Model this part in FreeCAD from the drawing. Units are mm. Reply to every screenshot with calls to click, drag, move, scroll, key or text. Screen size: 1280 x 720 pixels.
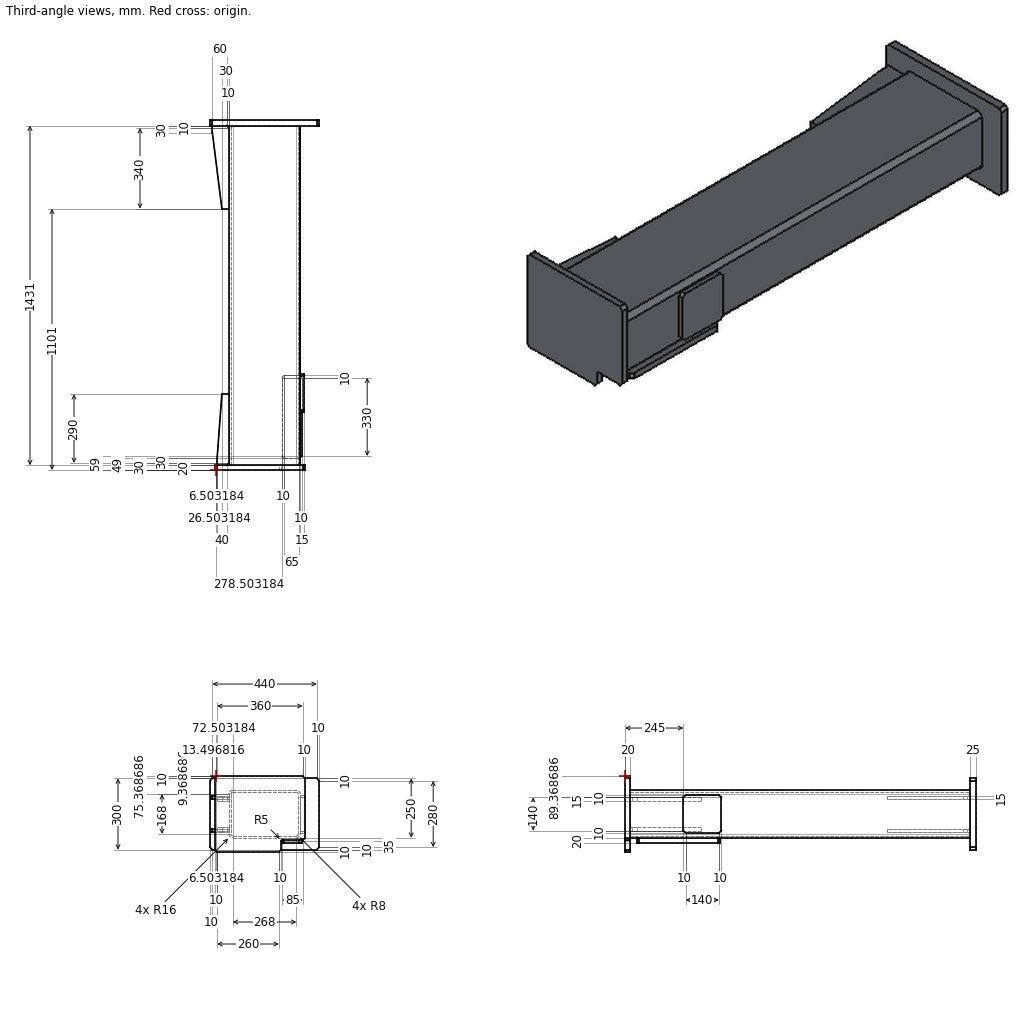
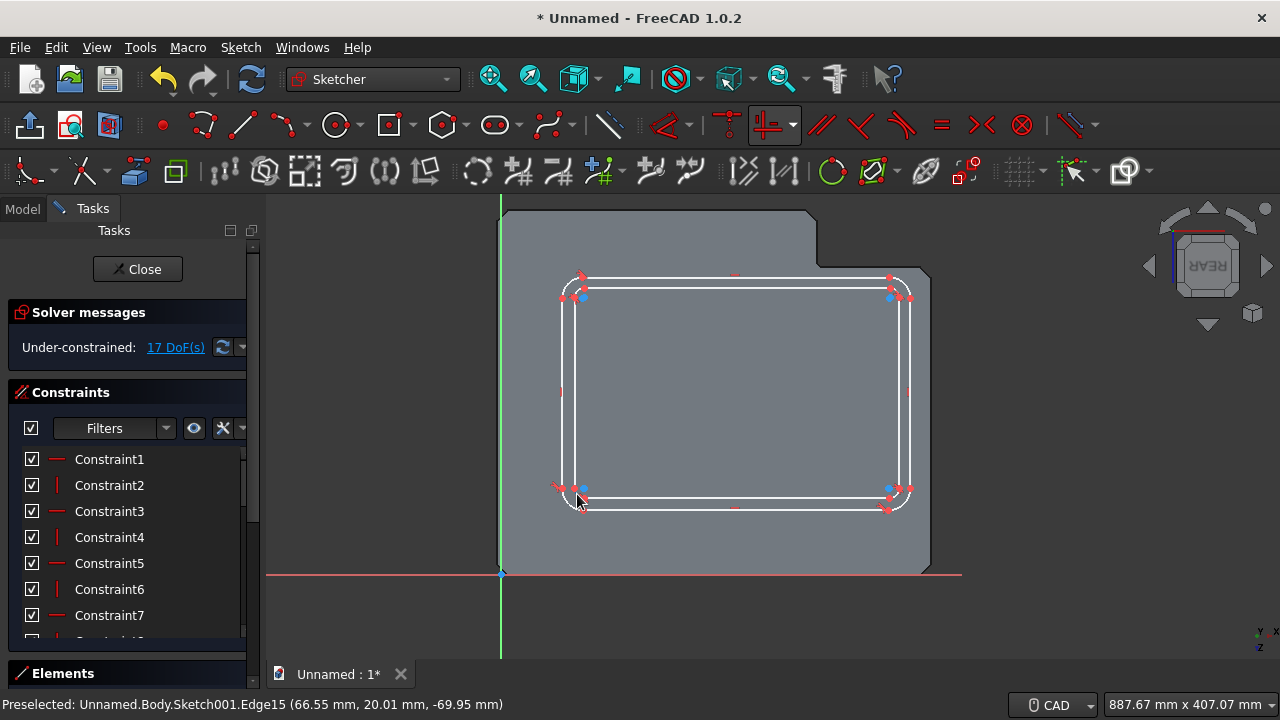
click(575, 431)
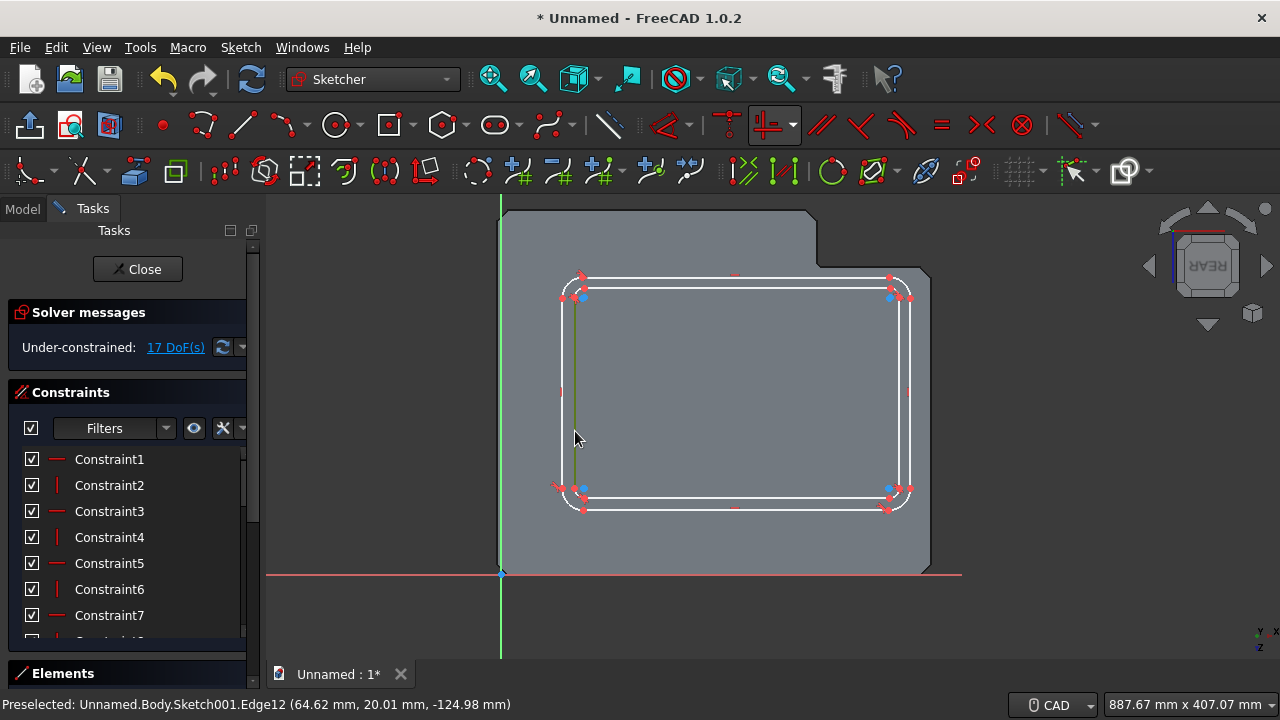
scroll(578, 291, up, 4)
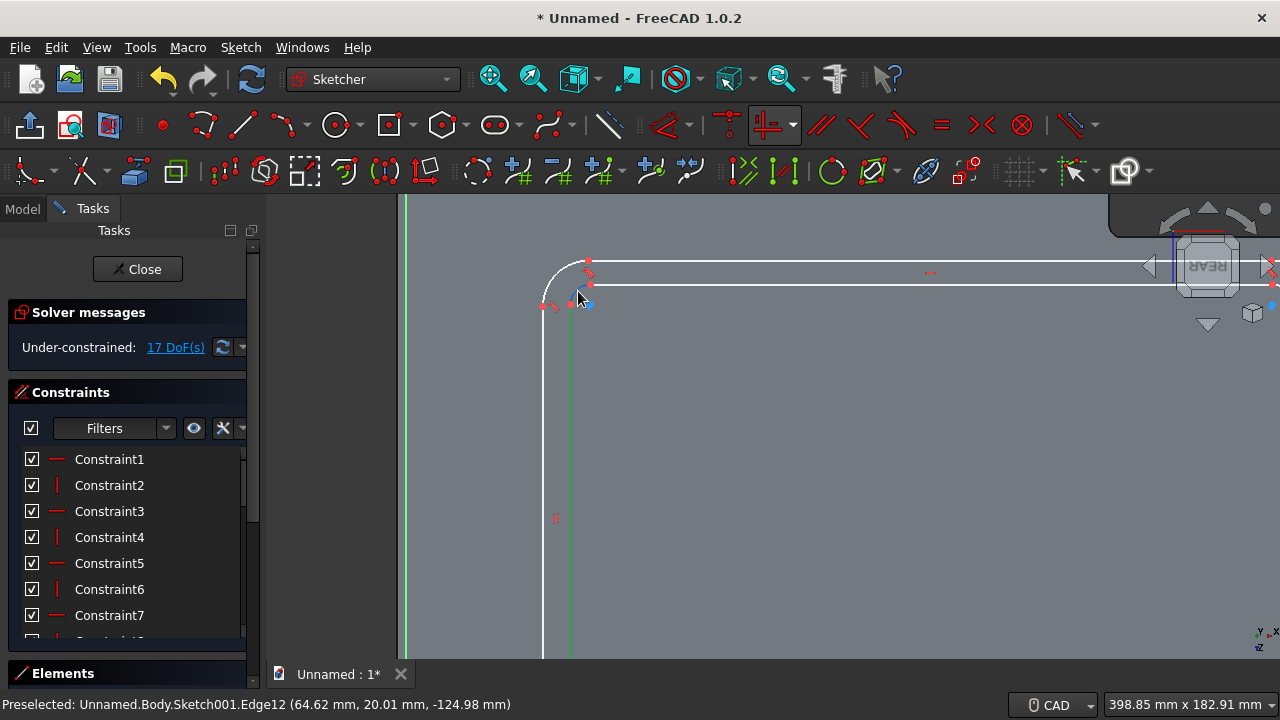
click(577, 290)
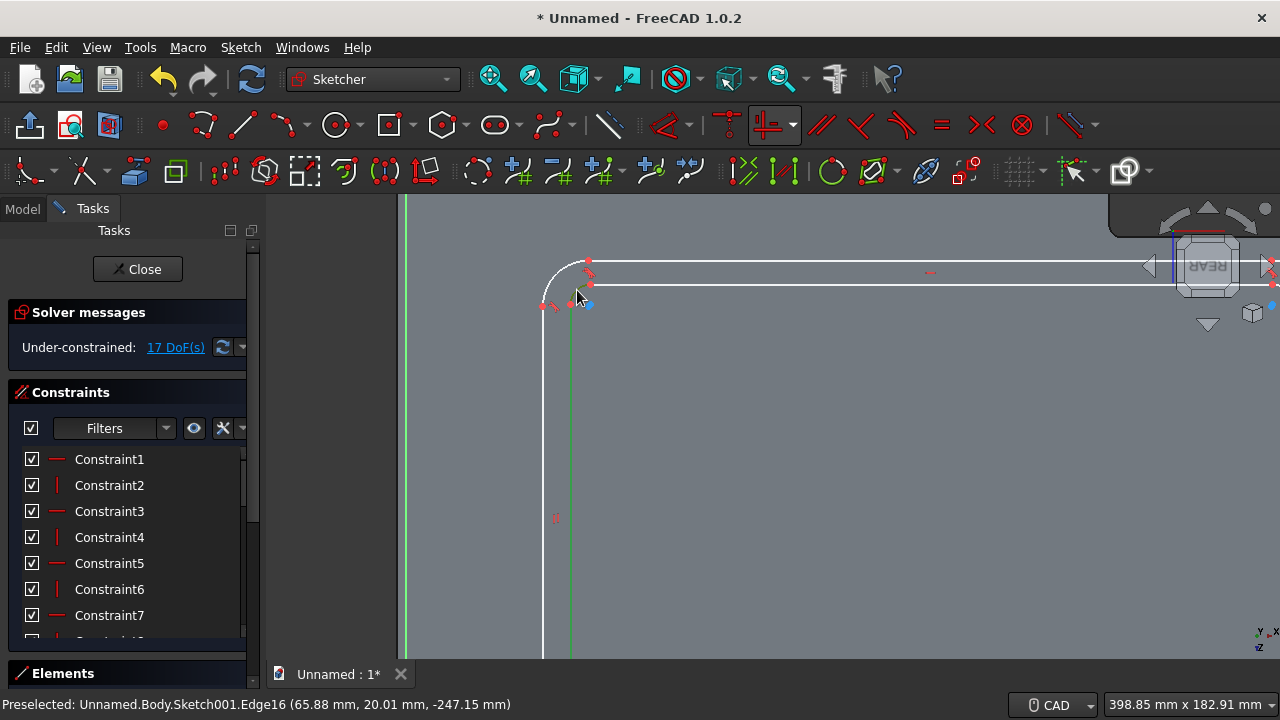
click(902, 126)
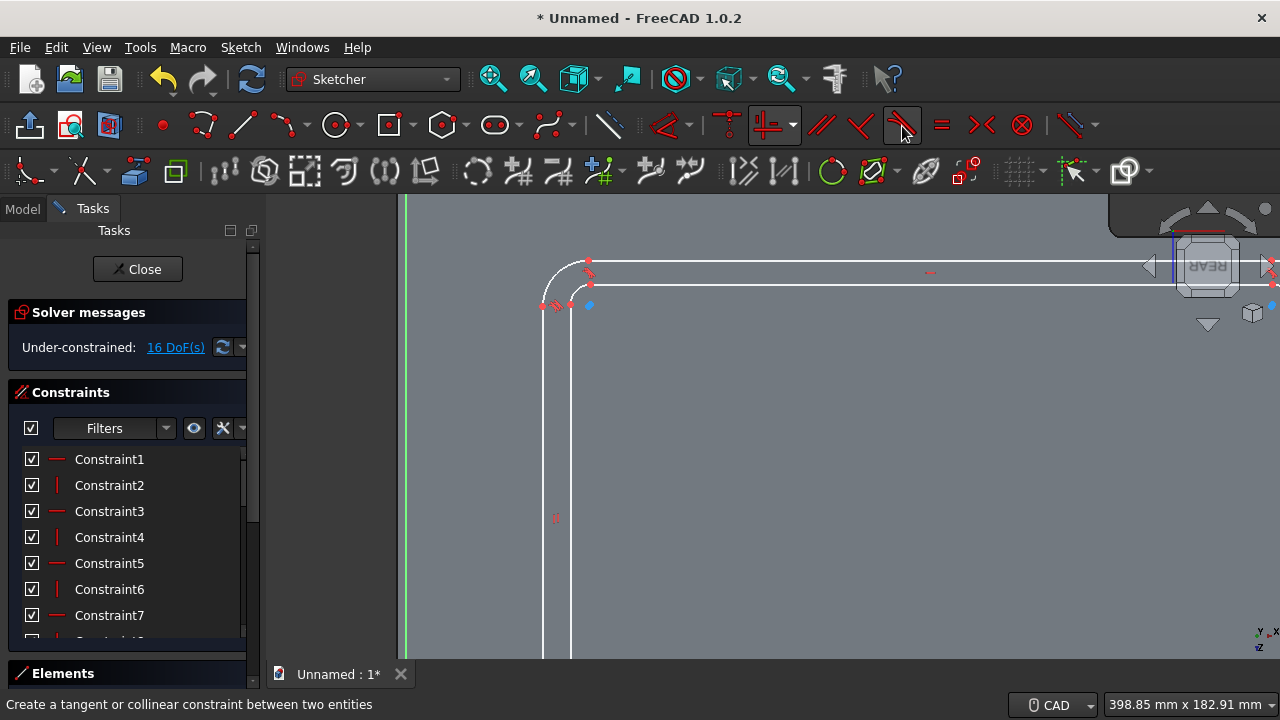
scroll(578, 291, down, 4)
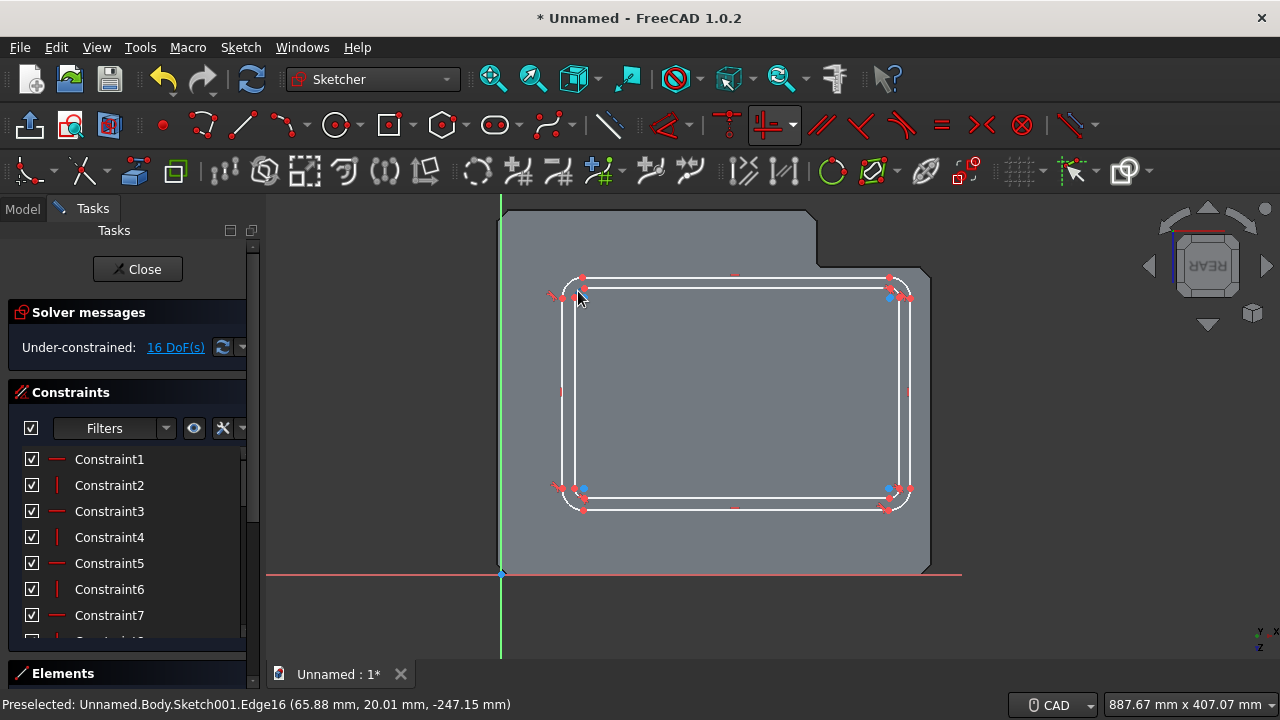
scroll(908, 289, up, 2)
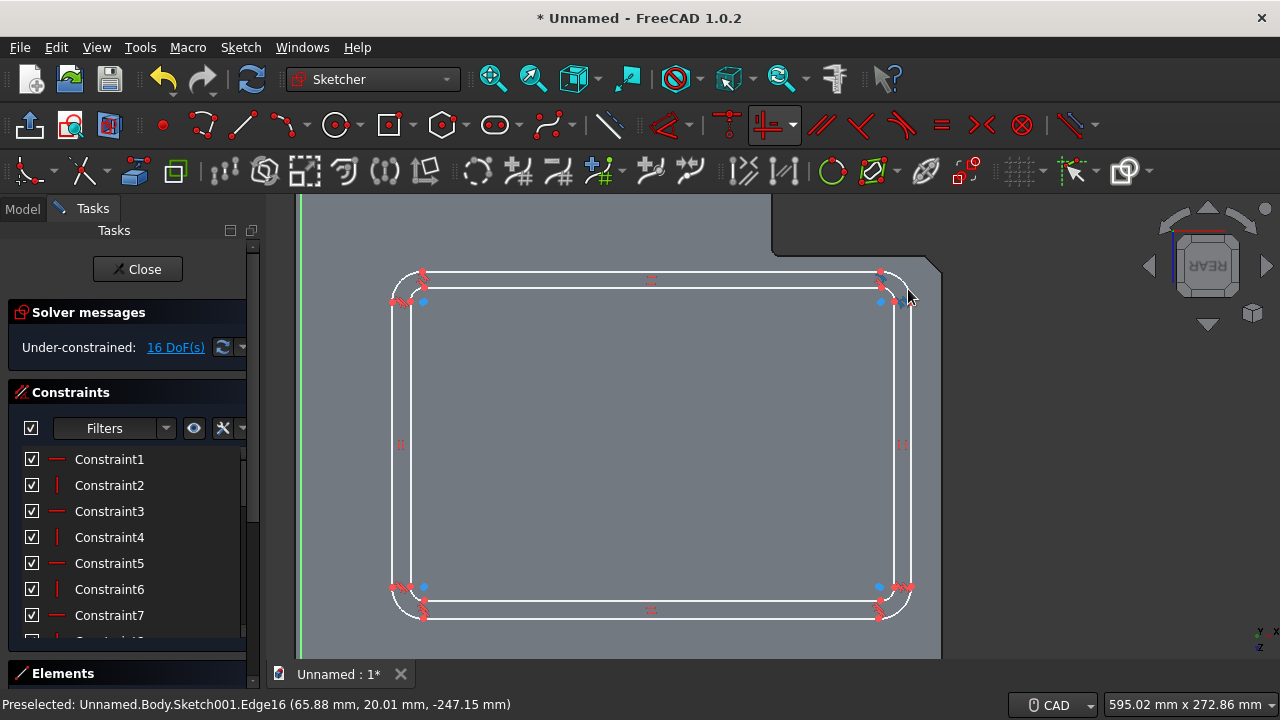
click(908, 289)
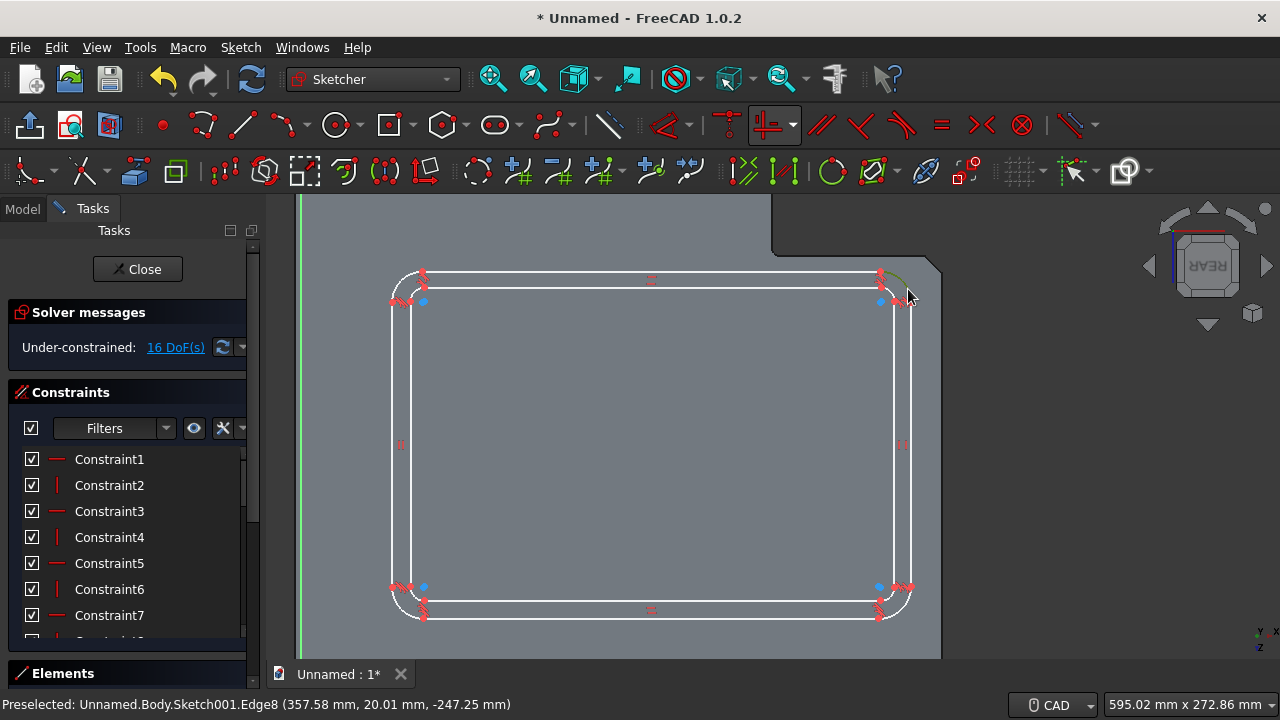
scroll(891, 292, up, 2)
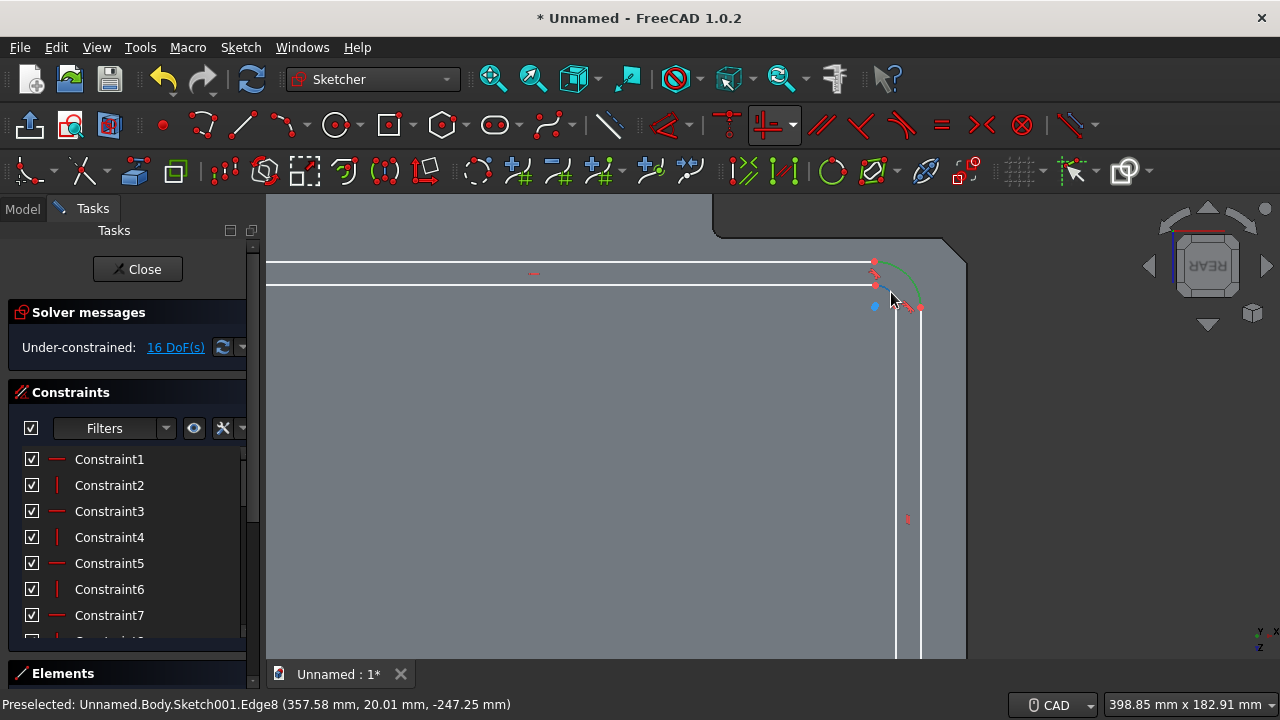
click(890, 291)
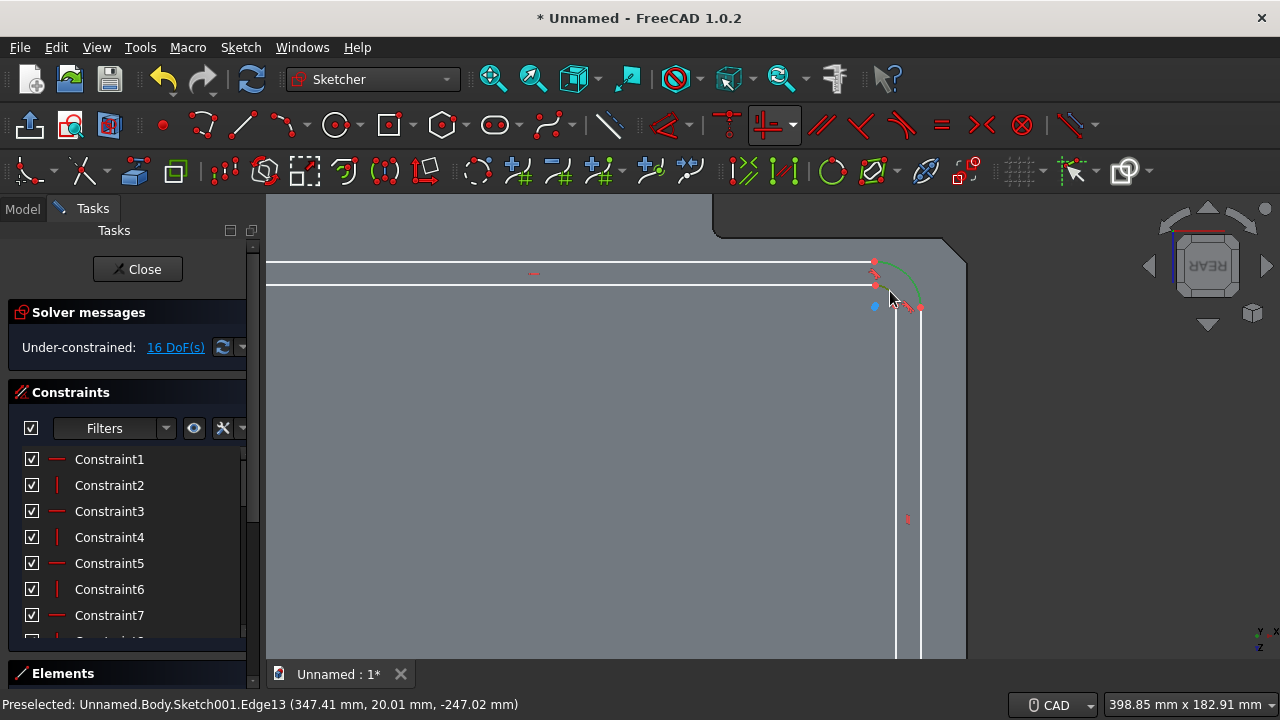
key(c)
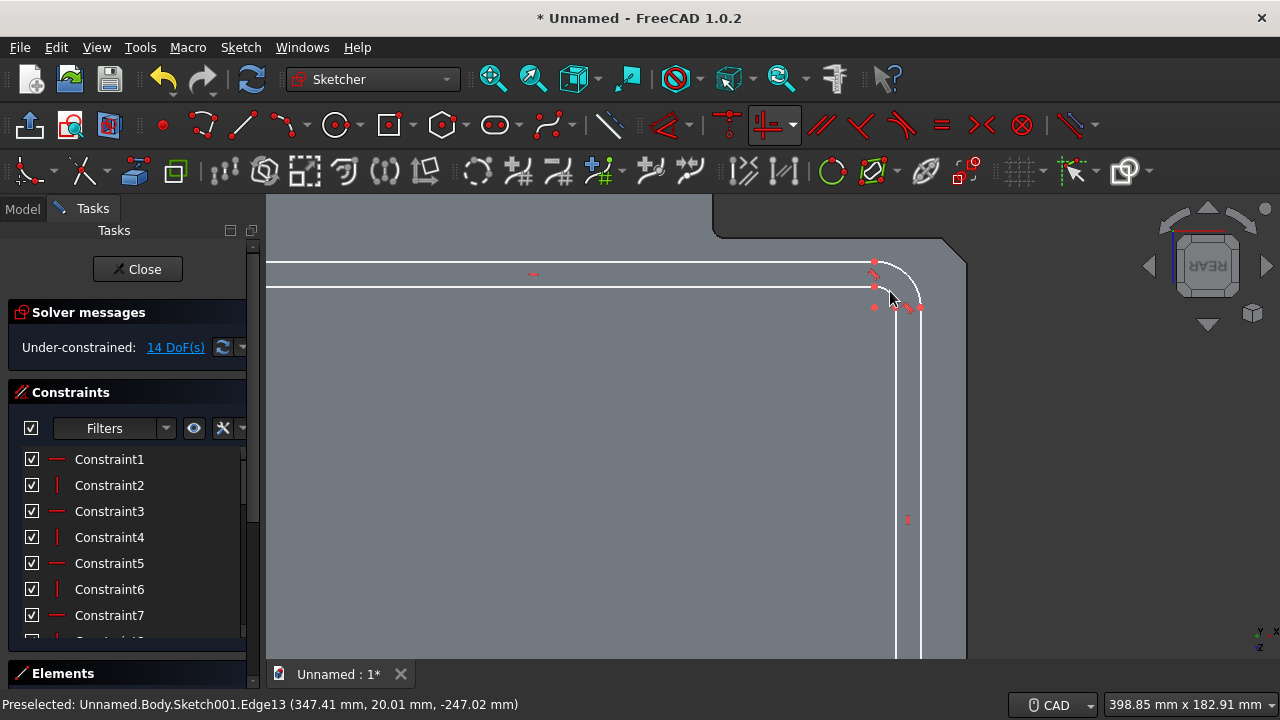
scroll(902, 290, down, 4)